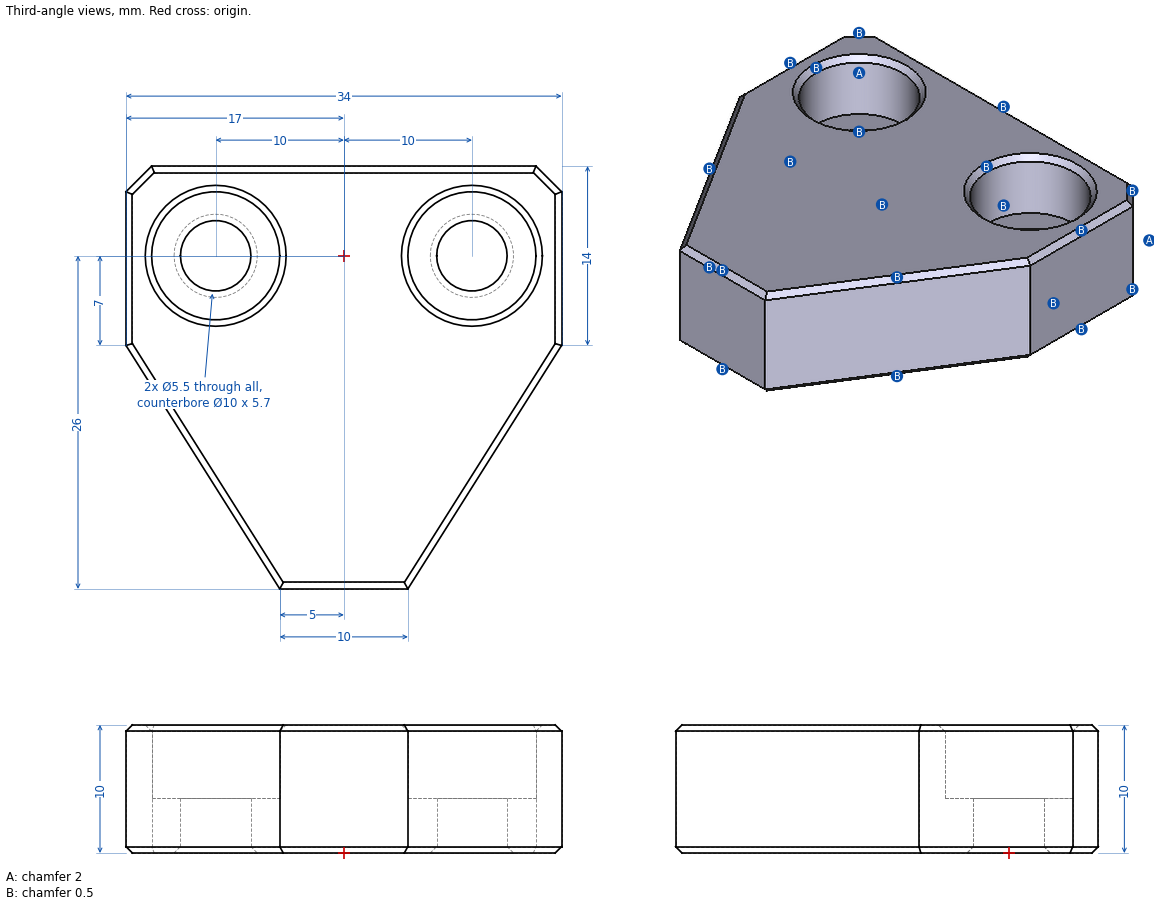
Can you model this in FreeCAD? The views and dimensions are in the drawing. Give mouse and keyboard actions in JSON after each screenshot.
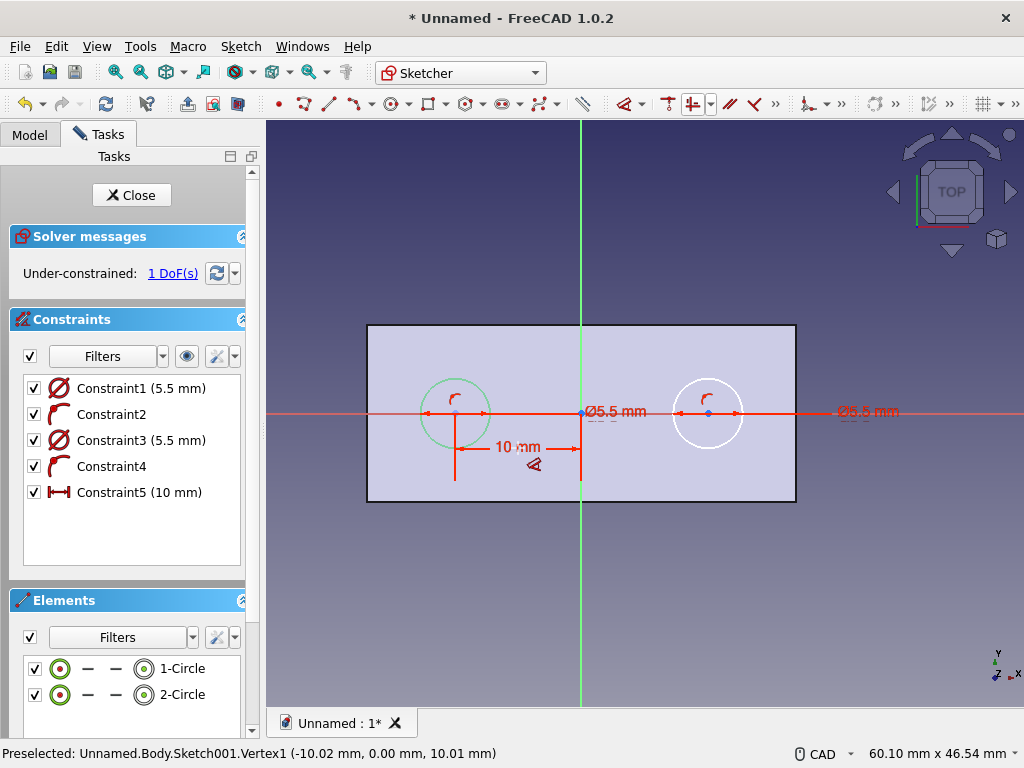
{"action": "left_click", "coordinate": [708, 414]}
{"action": "left_click", "coordinate": [645, 448]}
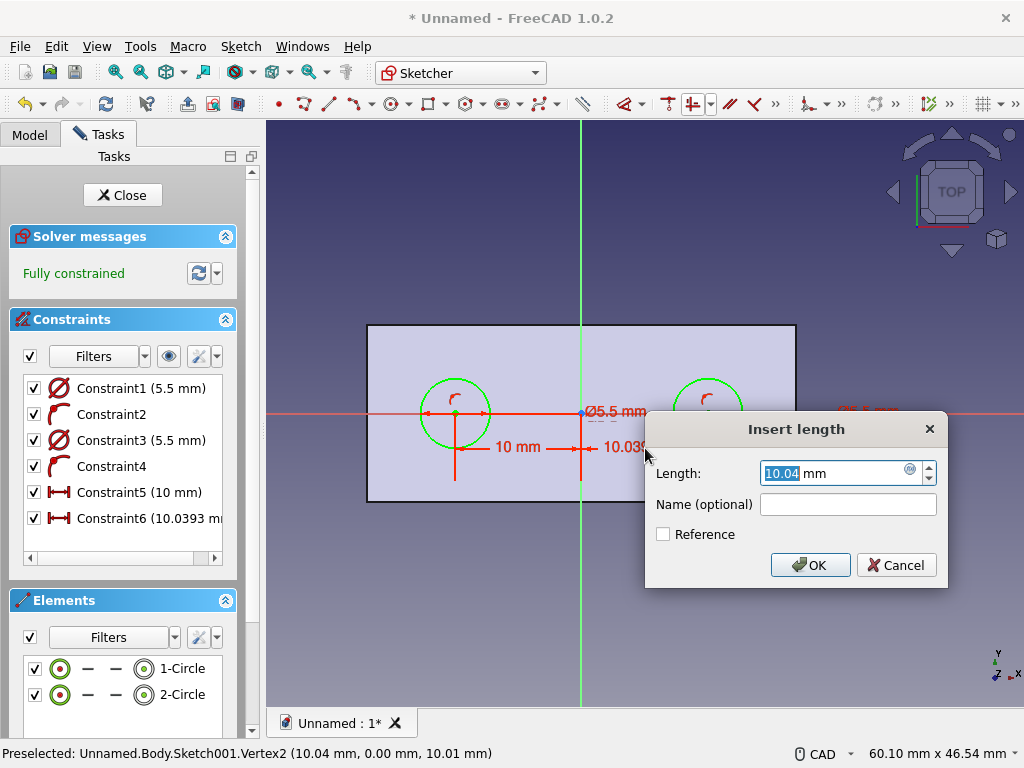
{"action": "type", "text": "10"}
{"action": "key", "text": "Return"}
{"action": "key", "text": "Escape"}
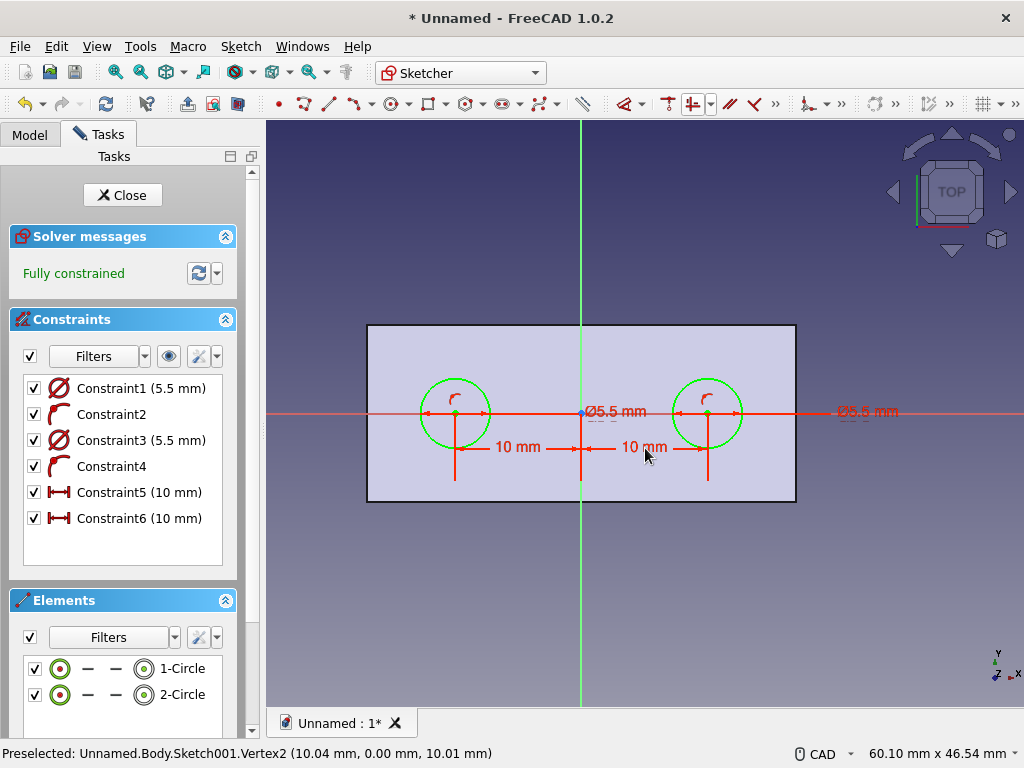
{"action": "left_click", "coordinate": [123, 195]}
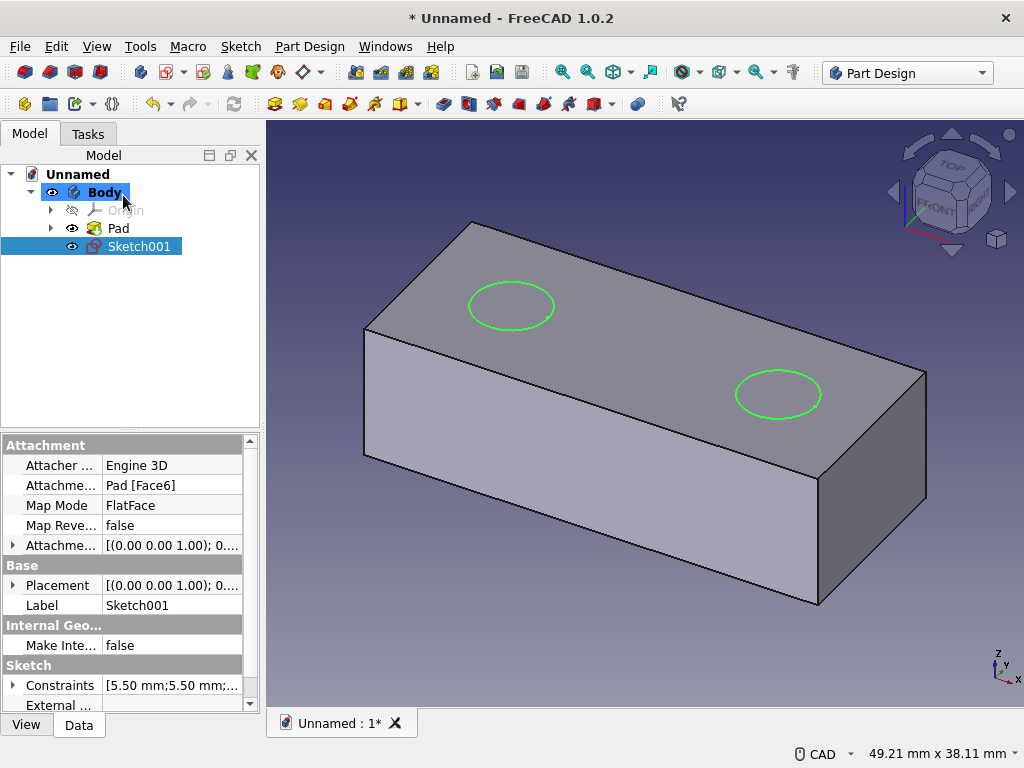
{"action": "left_click", "coordinate": [469, 104]}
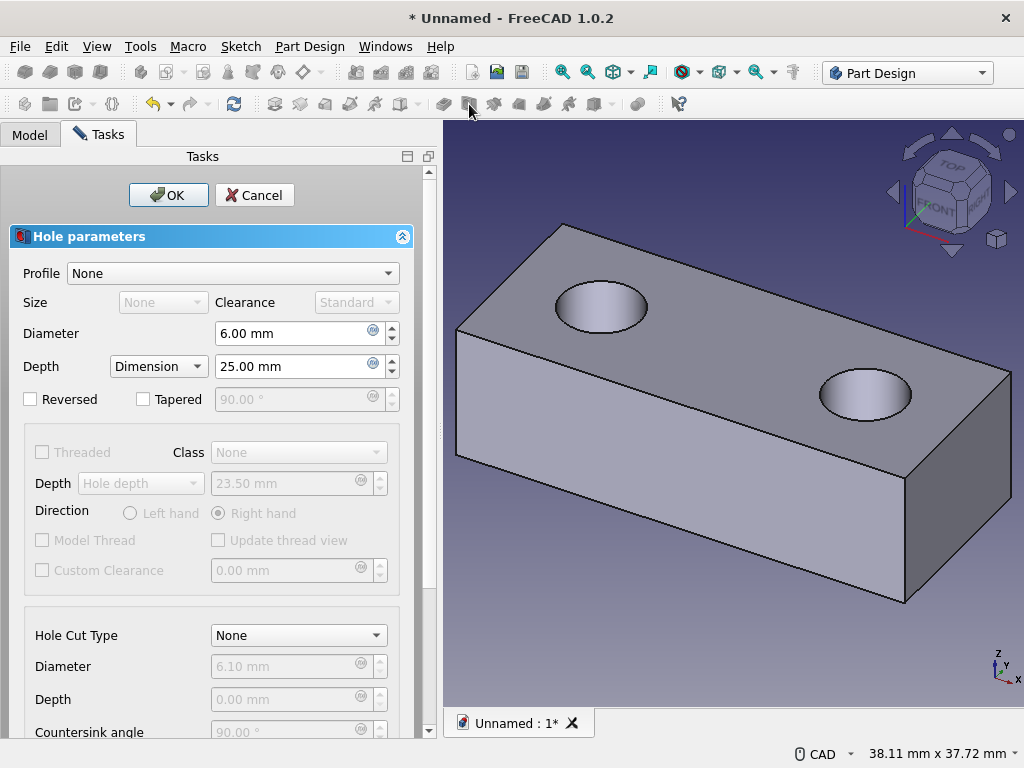
{"action": "triple_click", "coordinate": [300, 334]}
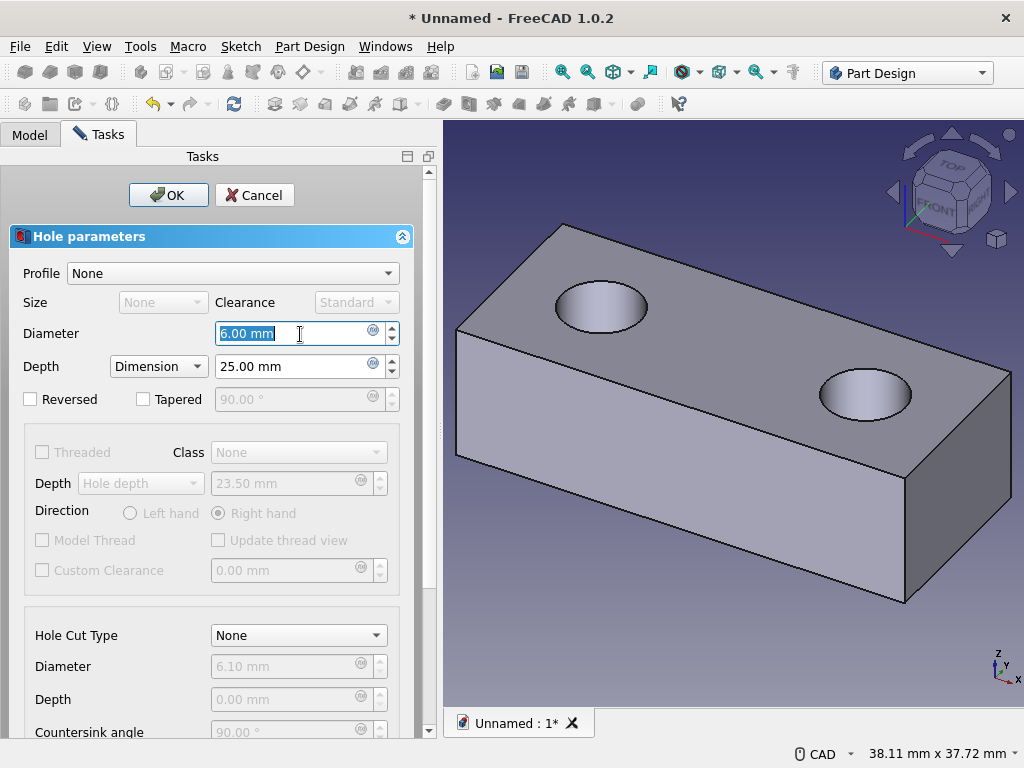
{"action": "type", "text": "5.5"}
{"action": "key", "text": "Tab"}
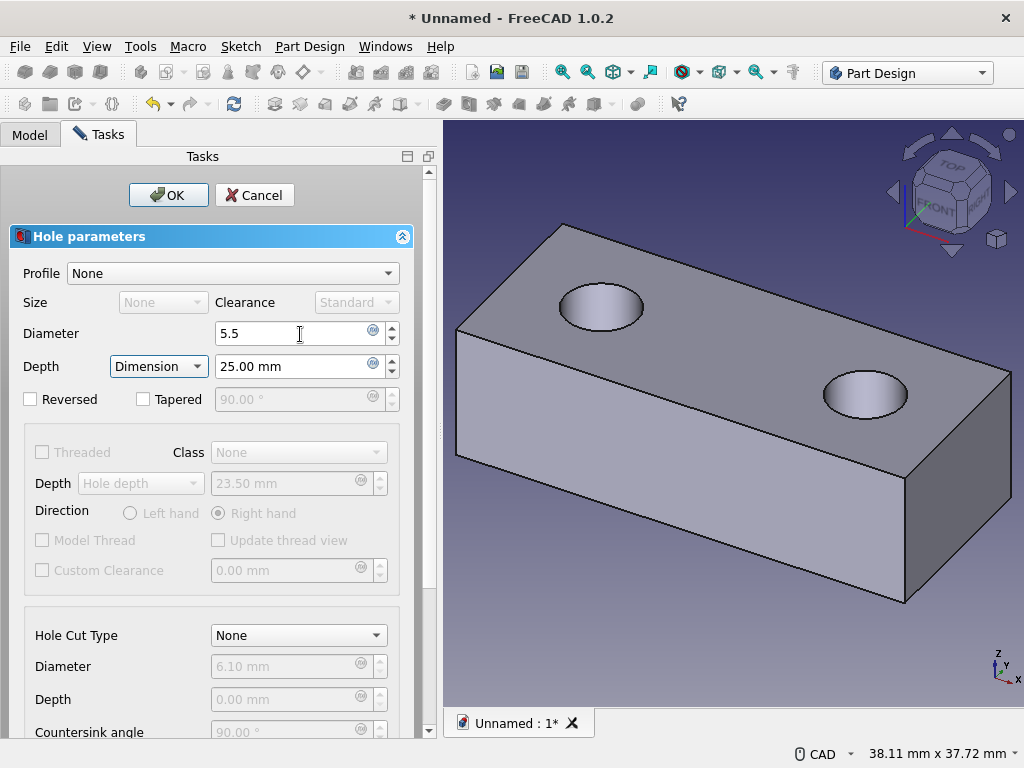
{"action": "left_click", "coordinate": [160, 366]}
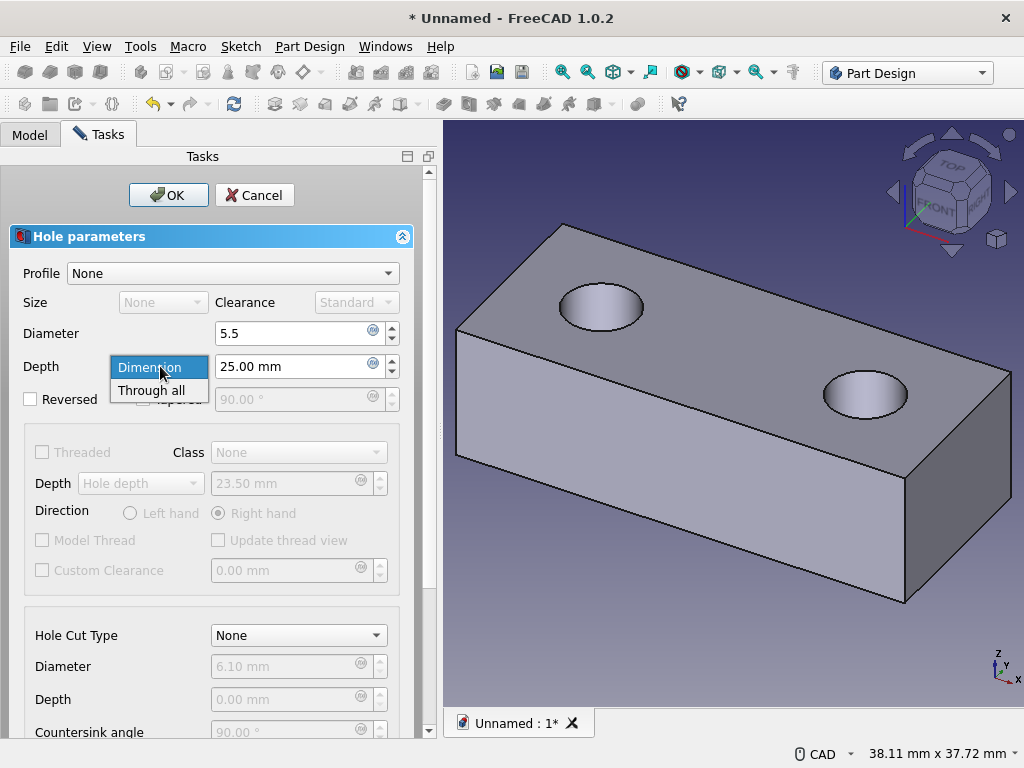
{"action": "left_click", "coordinate": [158, 390]}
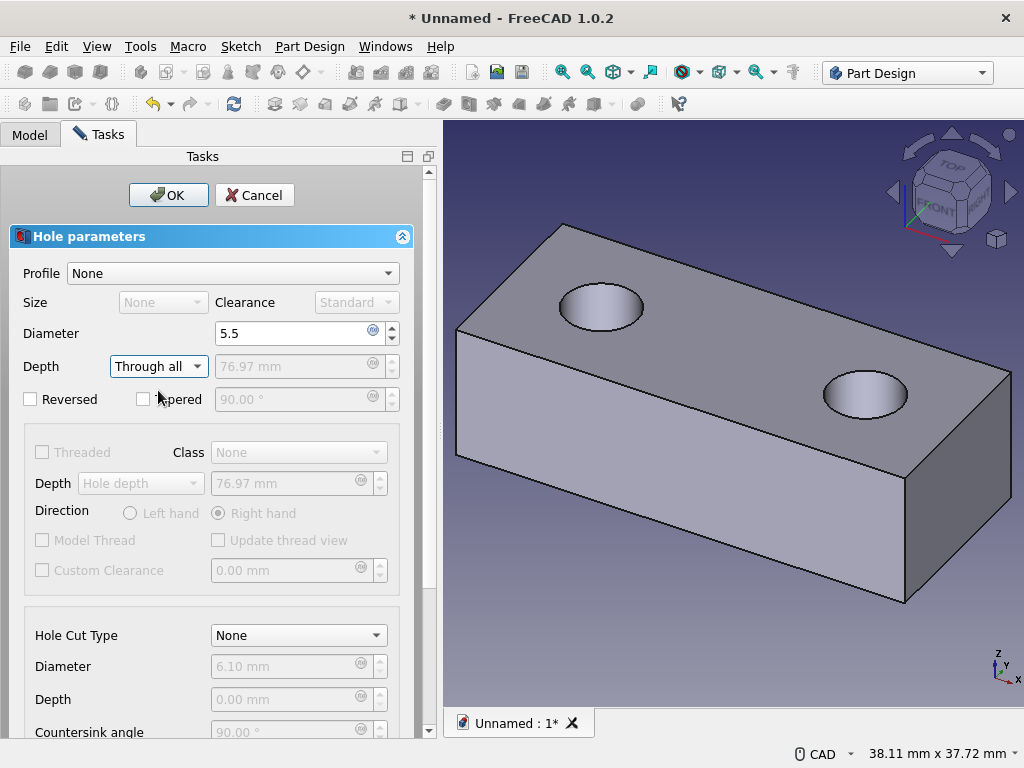
{"action": "left_click", "coordinate": [300, 636]}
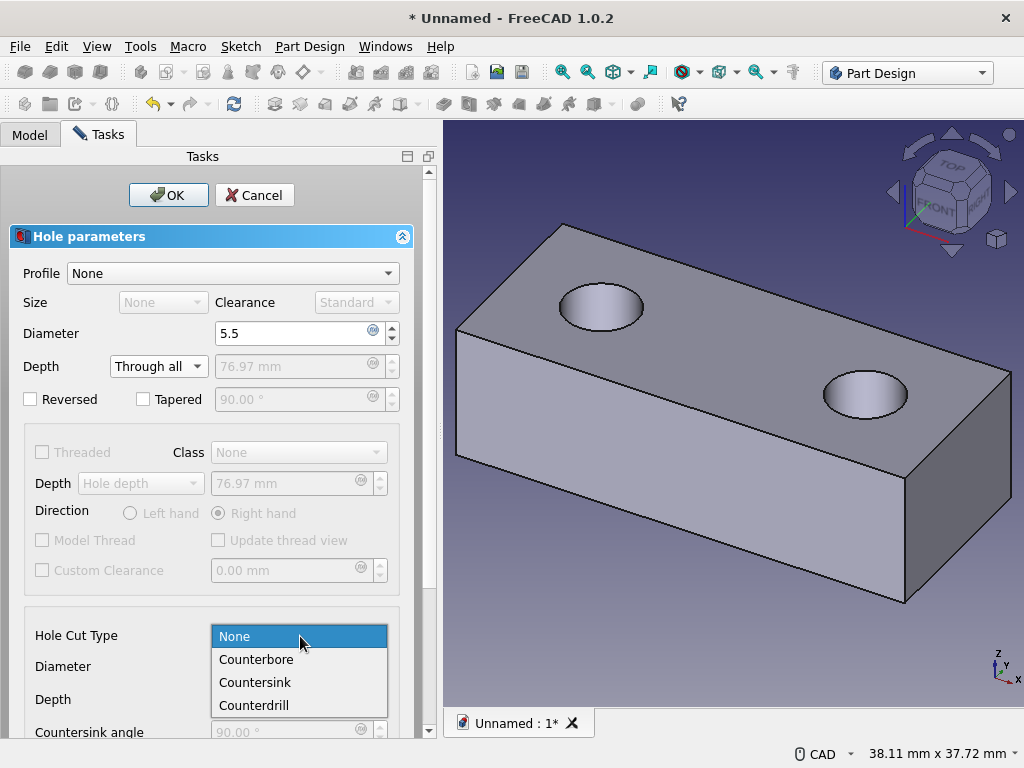
{"action": "left_click", "coordinate": [298, 660]}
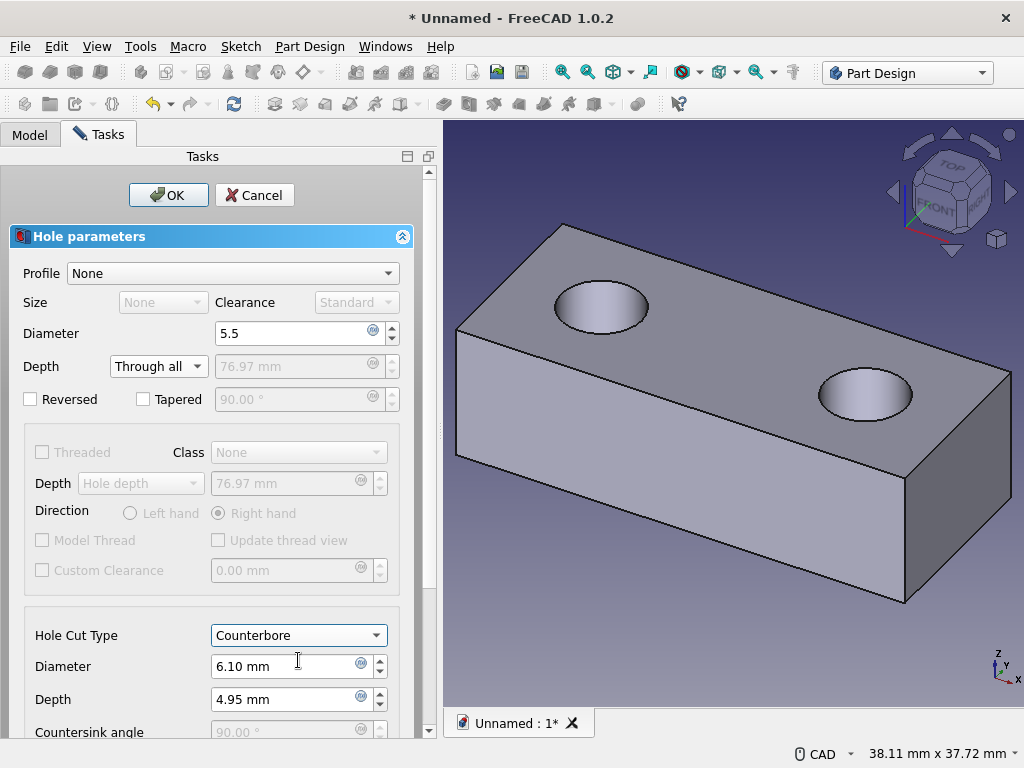
{"action": "triple_click", "coordinate": [292, 666]}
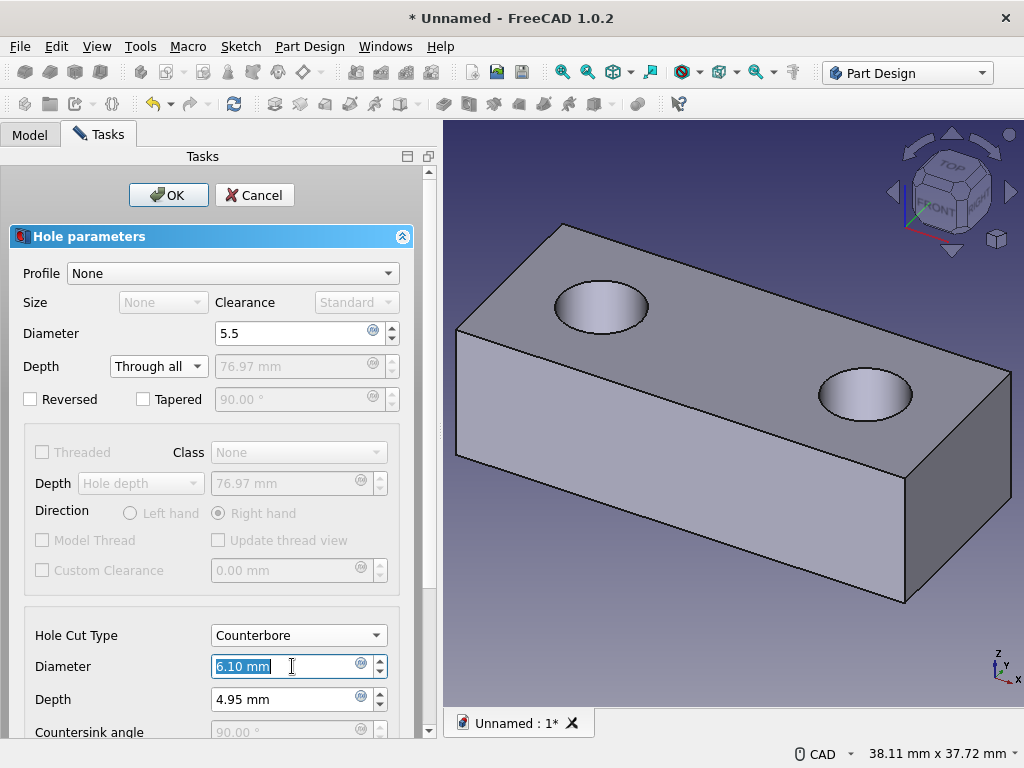
{"action": "type", "text": "10"}
{"action": "key", "text": "Tab"}